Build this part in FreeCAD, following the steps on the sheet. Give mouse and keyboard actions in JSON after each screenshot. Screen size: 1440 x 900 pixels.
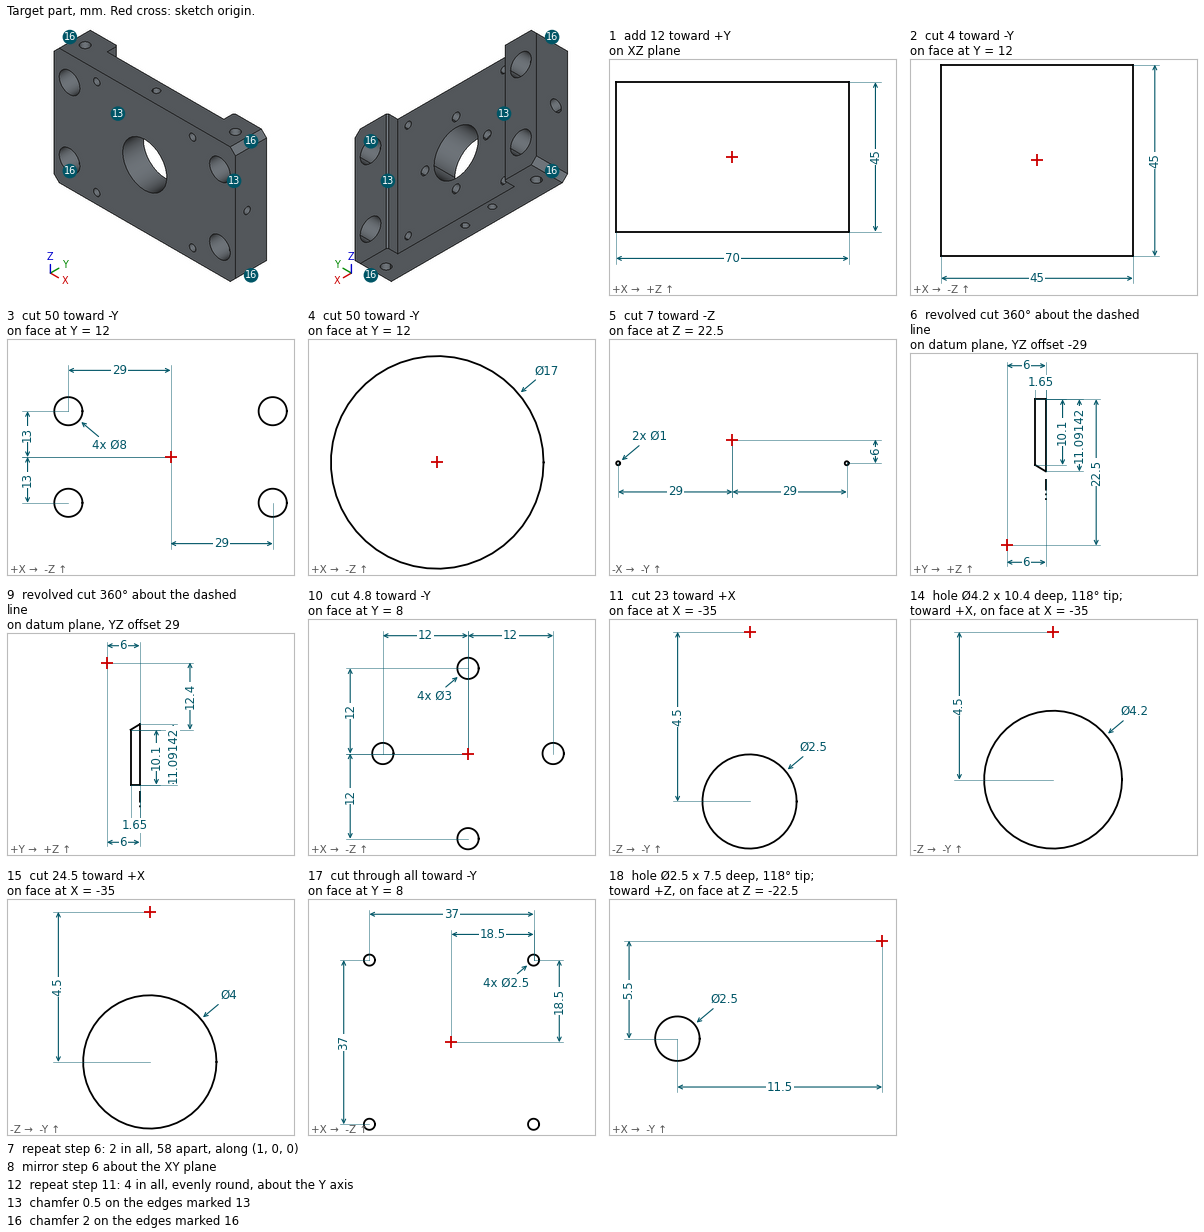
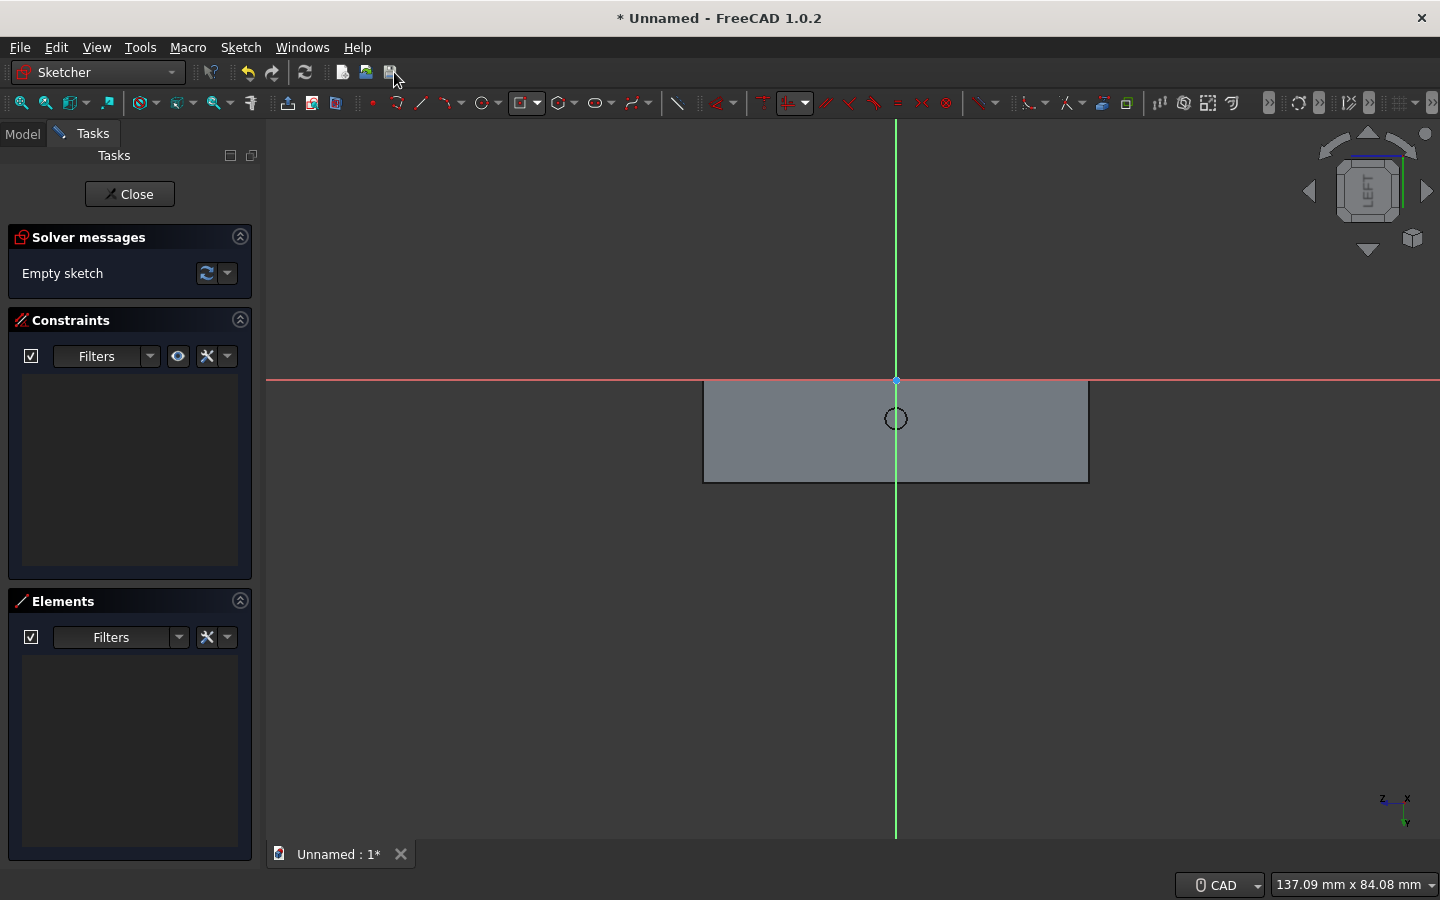
{"action": "scroll", "coordinate": [910, 400], "scroll_direction": "up", "scroll_amount": 11}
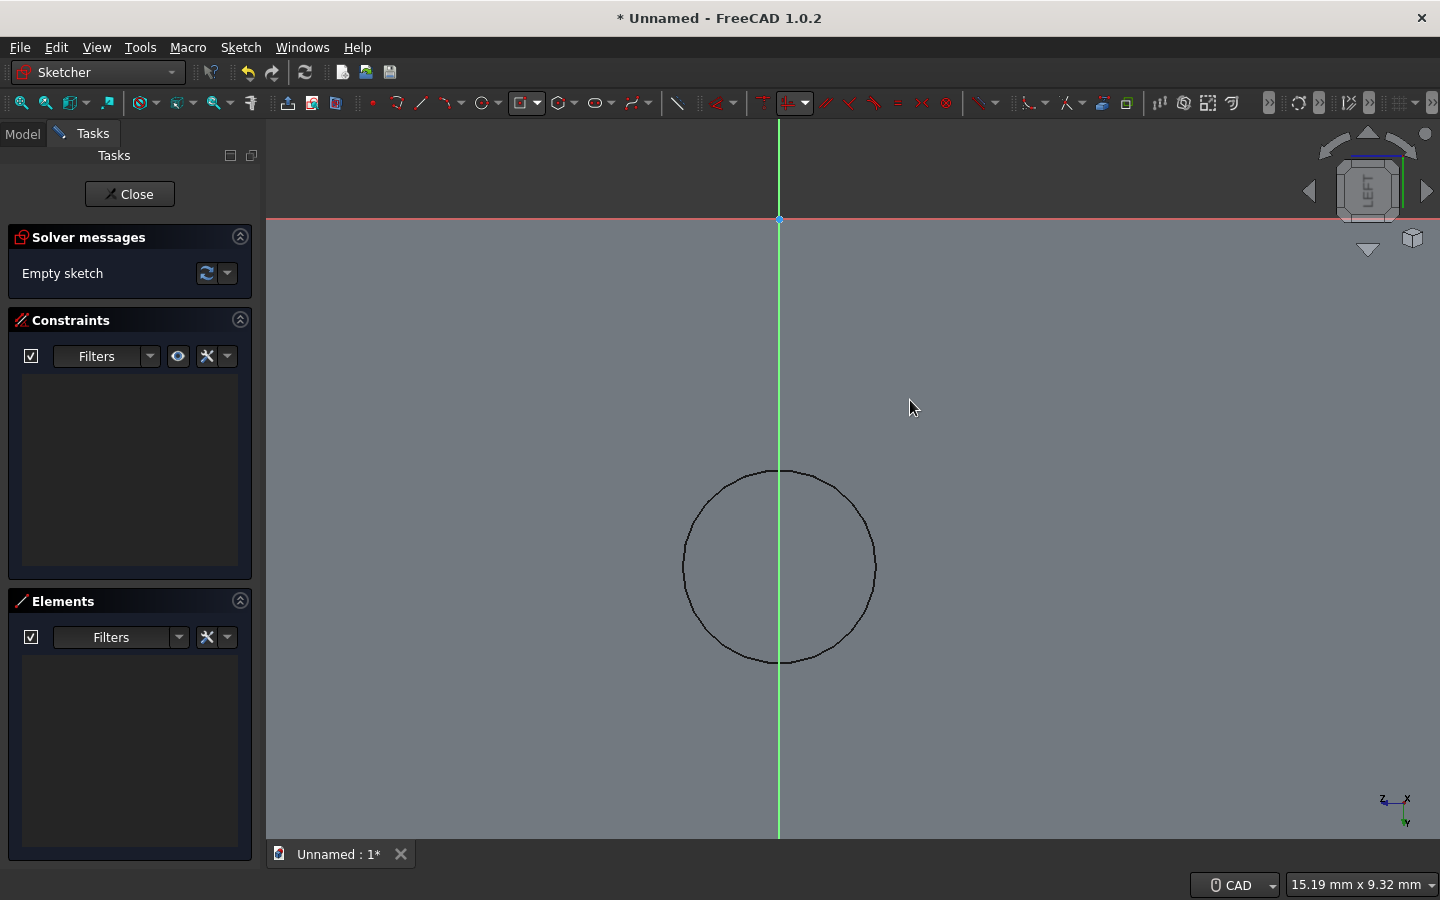
{"action": "left_click", "coordinate": [482, 104]}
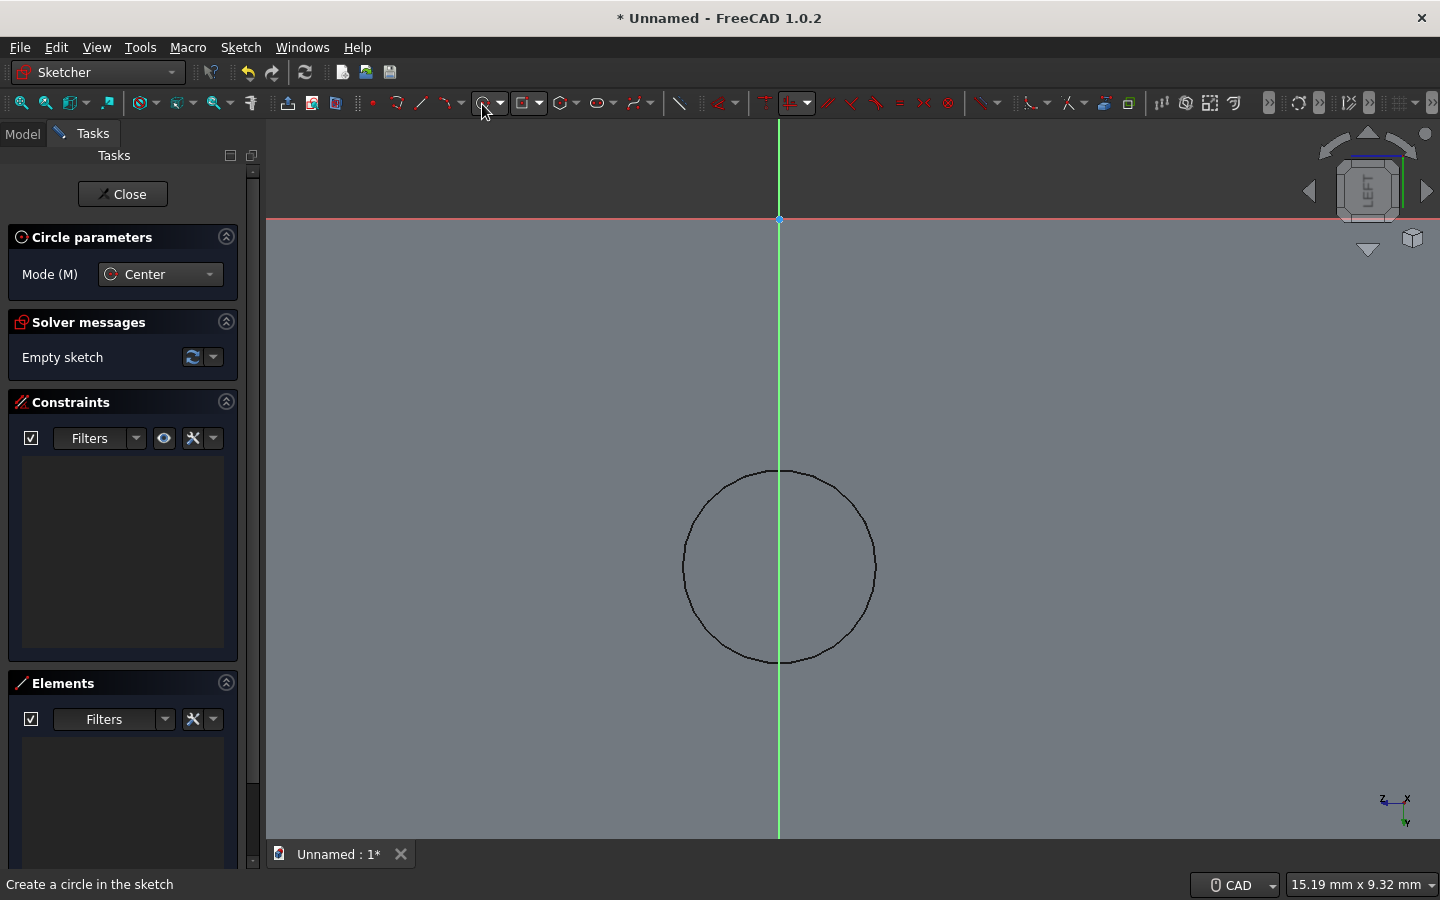
{"action": "left_click", "coordinate": [779, 567]}
{"action": "mouse_move", "coordinate": [894, 452]}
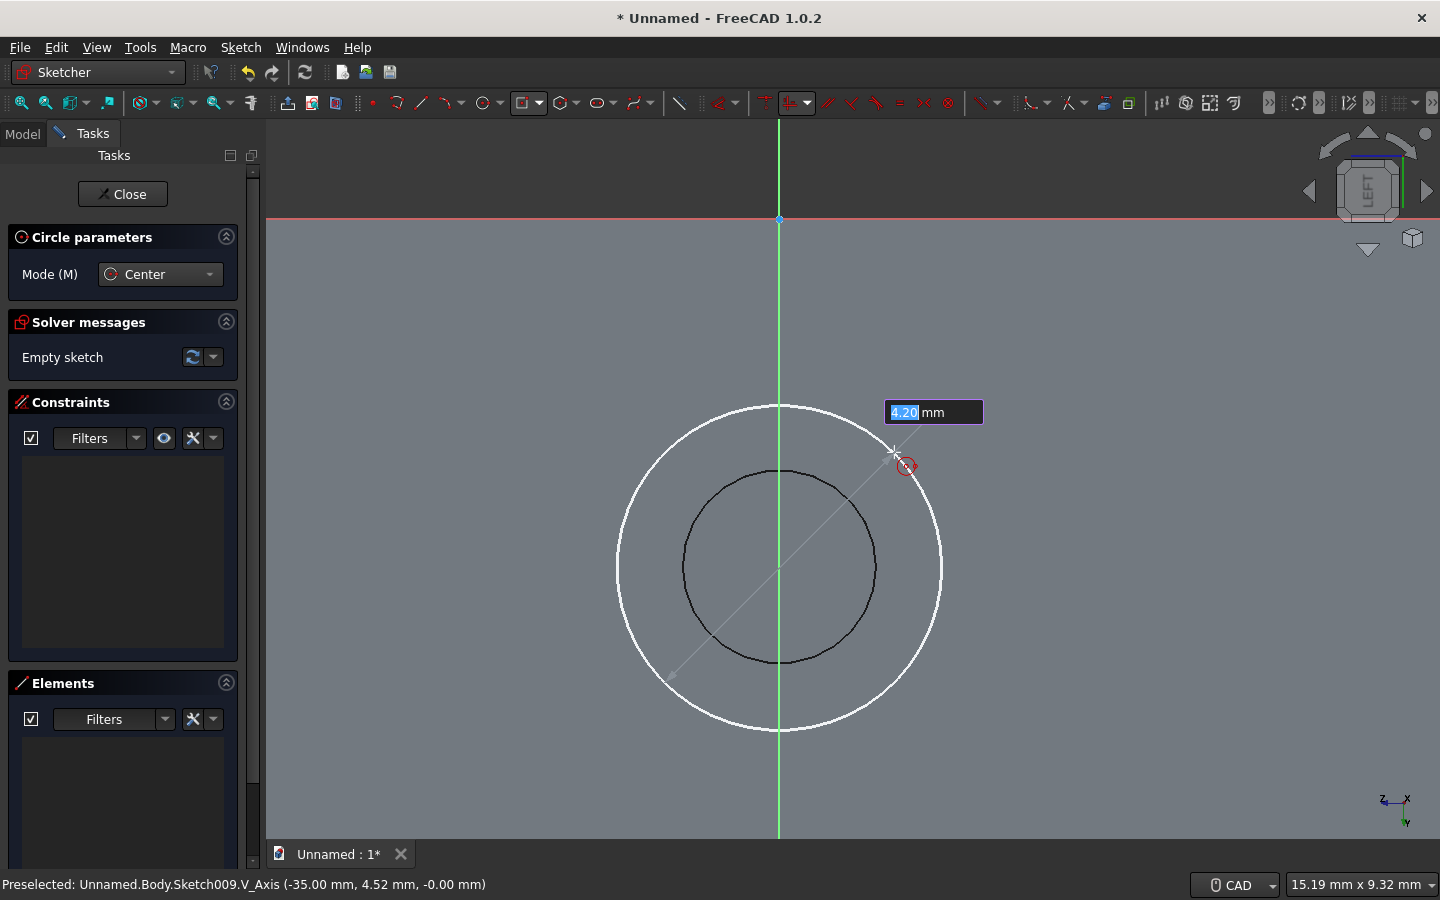
{"action": "type", "text": "4.2"}
{"action": "key", "text": "Return"}
{"action": "key", "text": "Escape"}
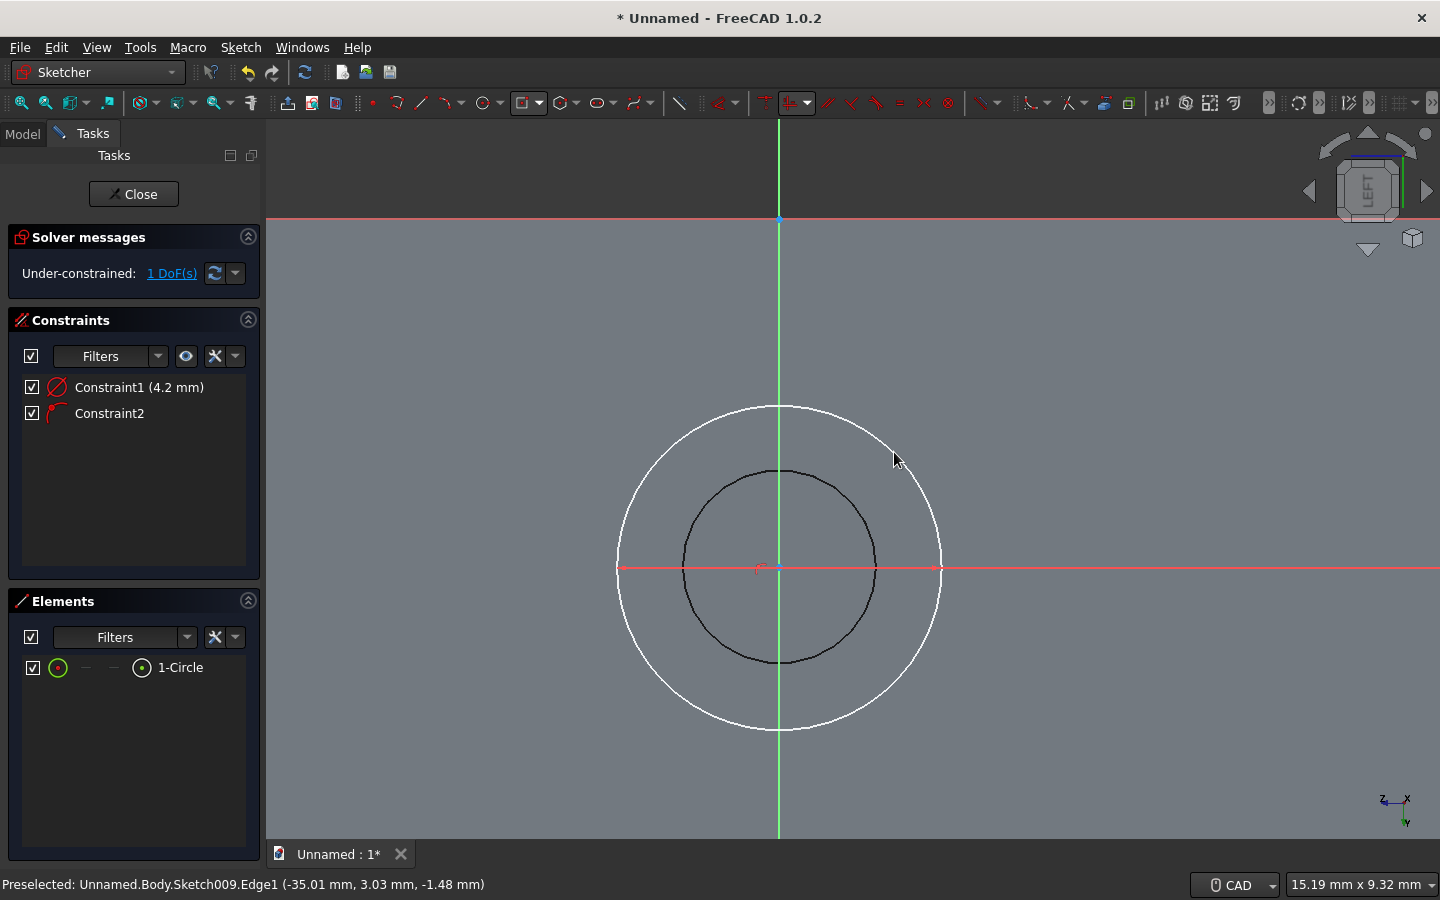
{"action": "left_click", "coordinate": [718, 104]}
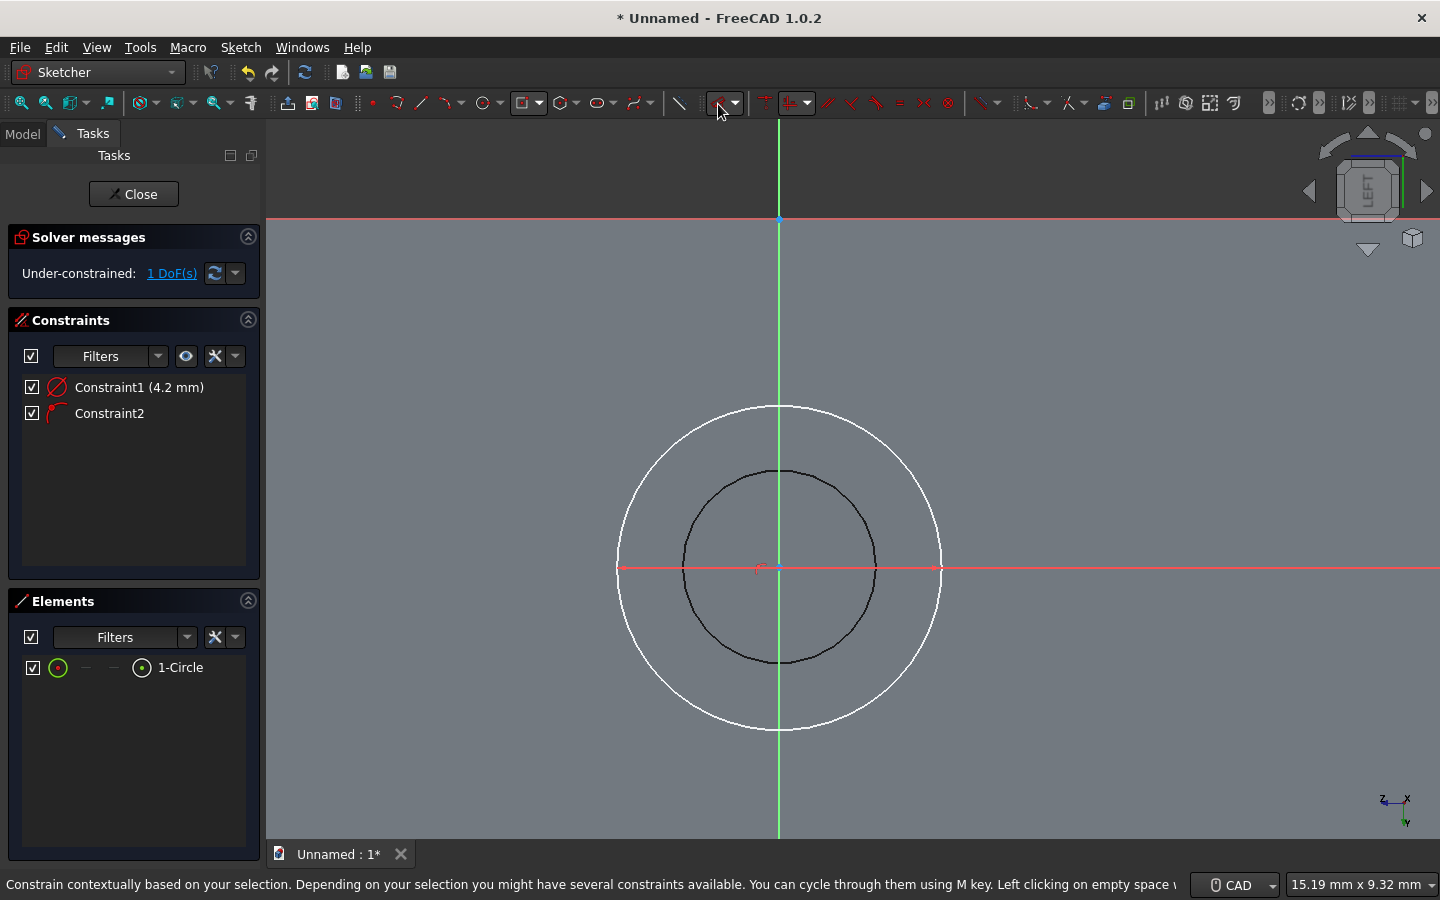
{"action": "left_click", "coordinate": [779, 568]}
{"action": "left_click", "coordinate": [813, 394]}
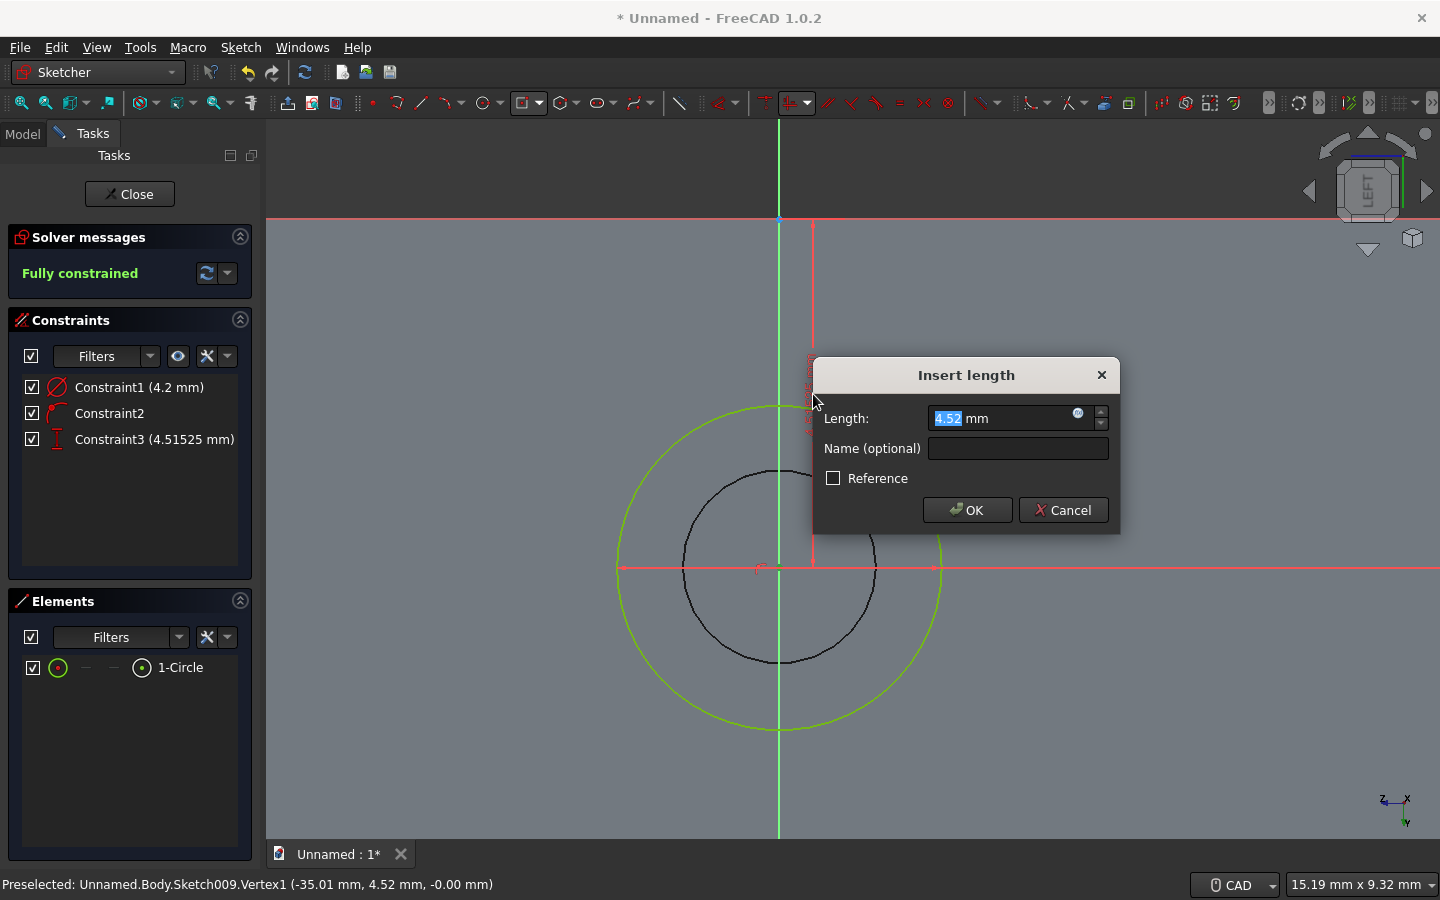
{"action": "type", "text": "4.5"}
{"action": "key", "text": "Return"}
{"action": "key", "text": "Escape"}